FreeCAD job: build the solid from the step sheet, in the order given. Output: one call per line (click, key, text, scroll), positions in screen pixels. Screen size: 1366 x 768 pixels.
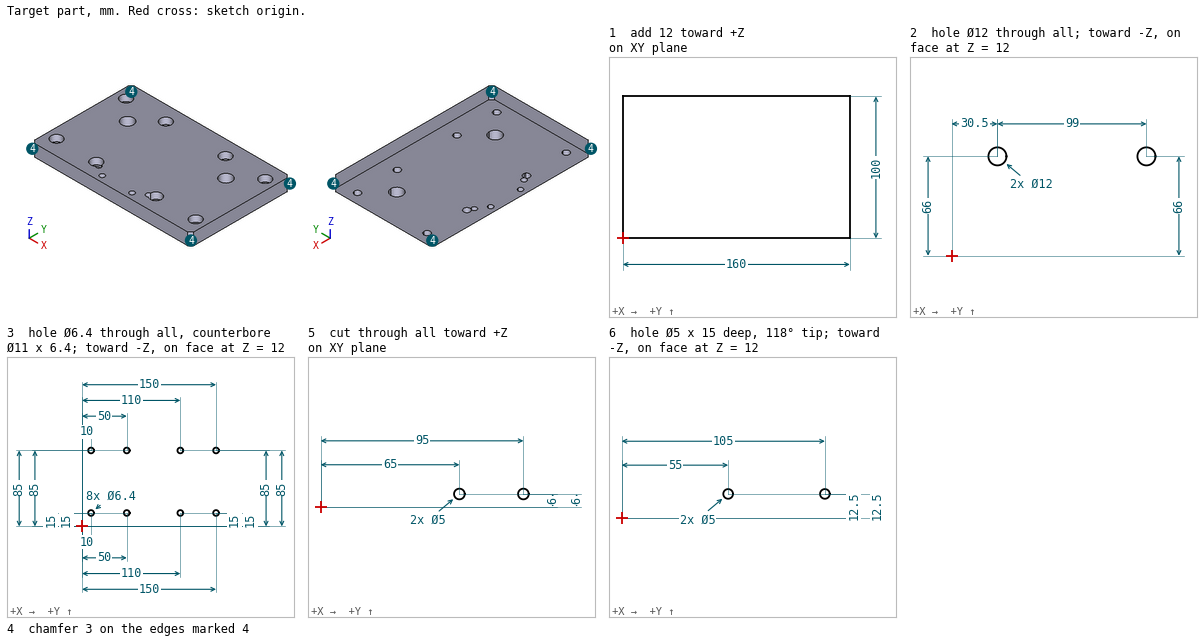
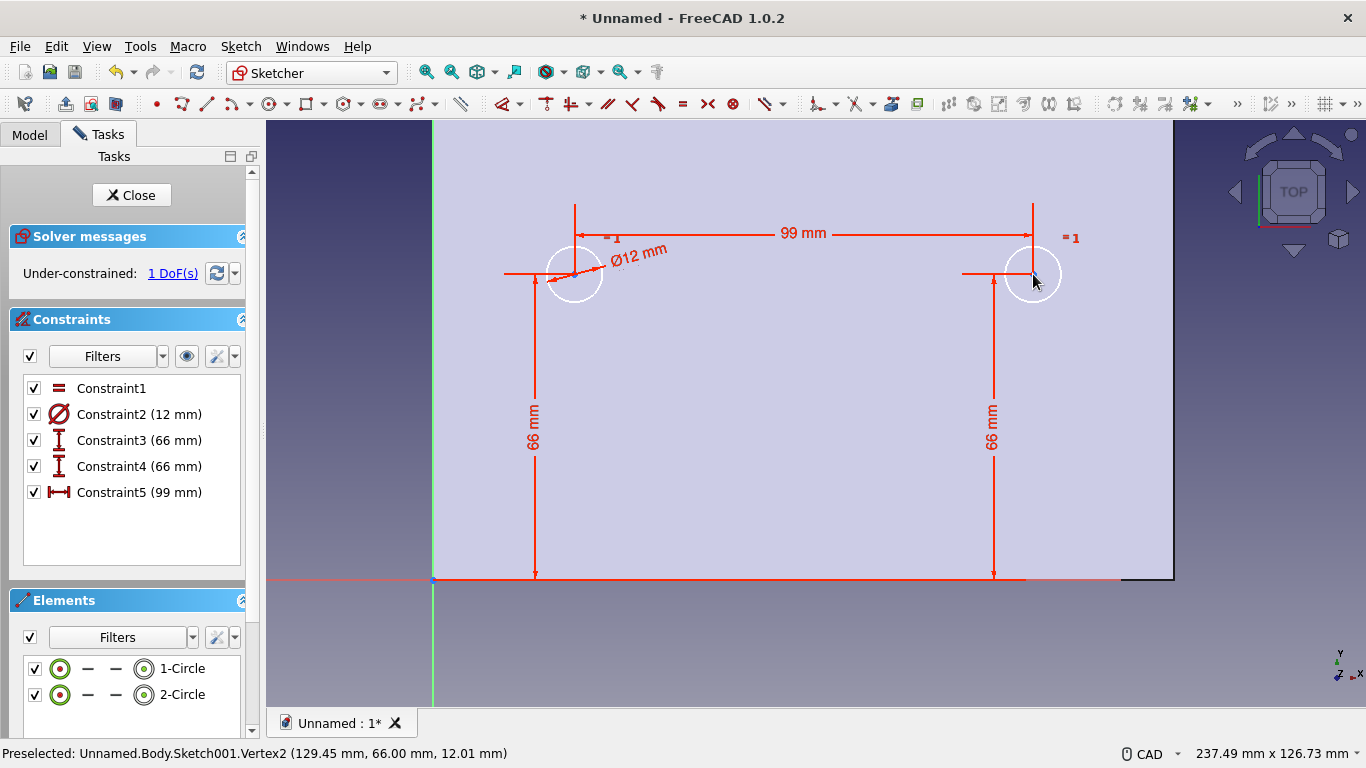
click(575, 274)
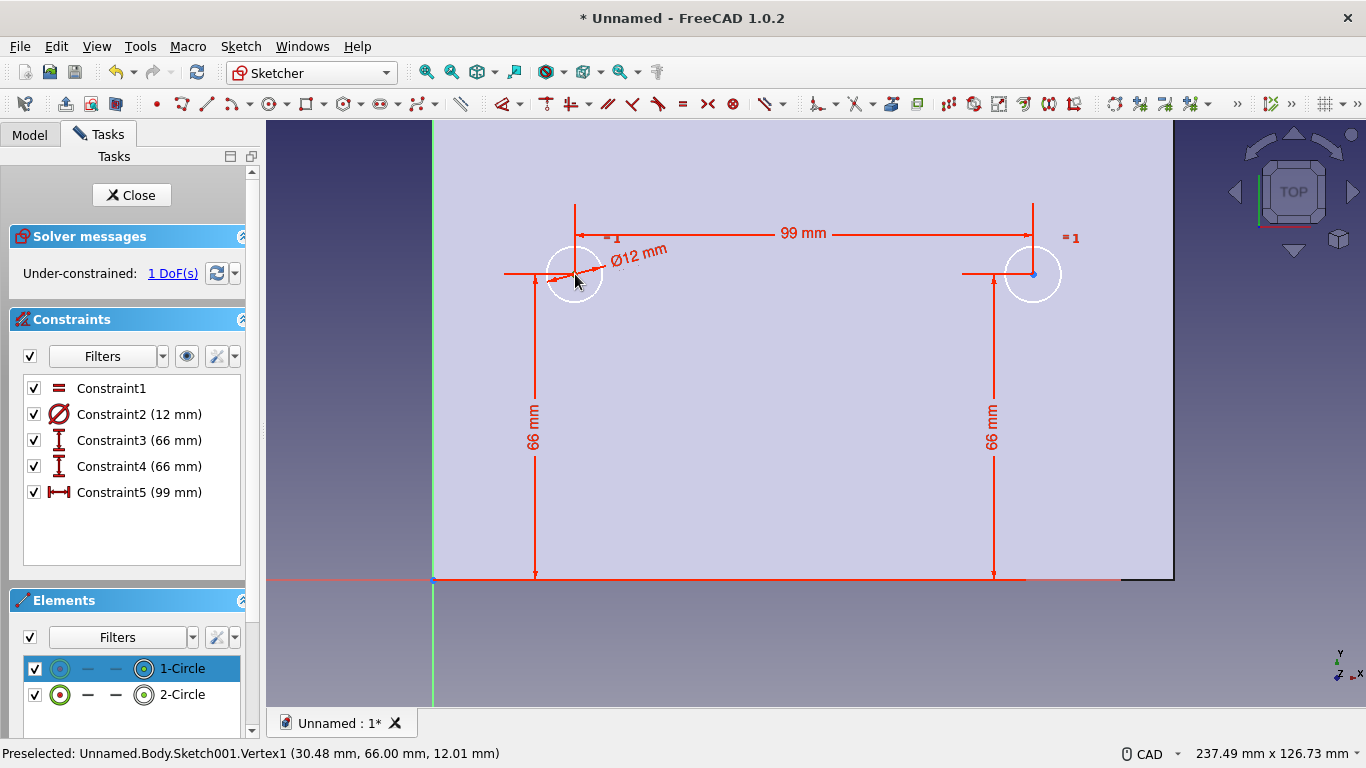
key(l)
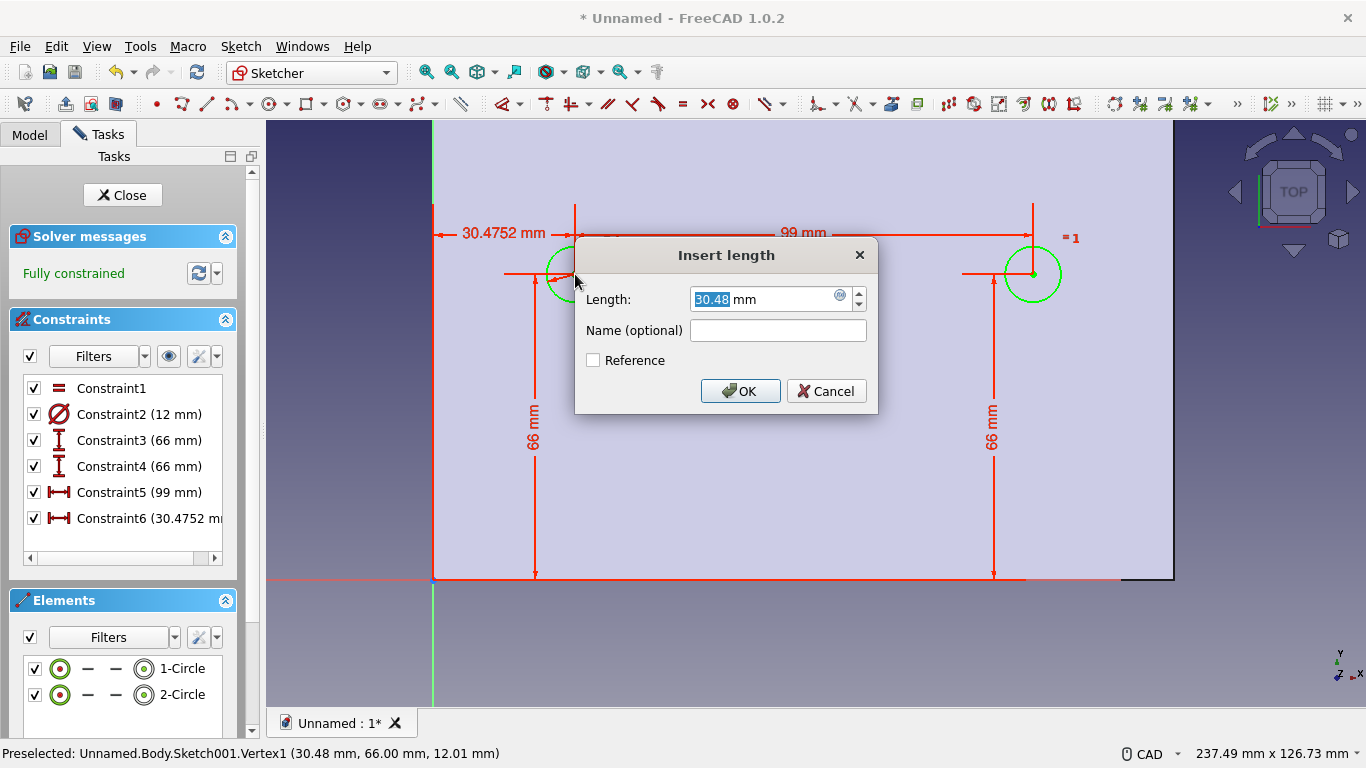
text(30.5)
key(Return)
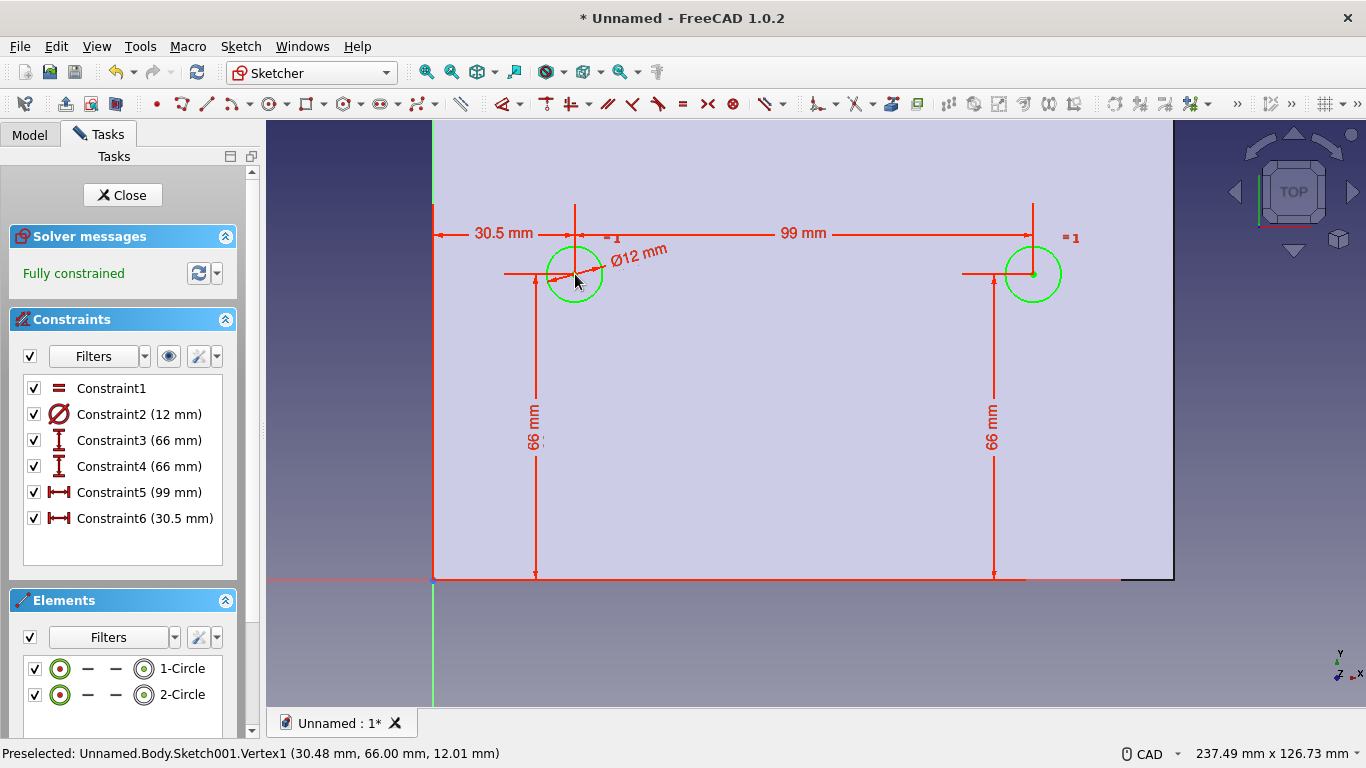
click(123, 195)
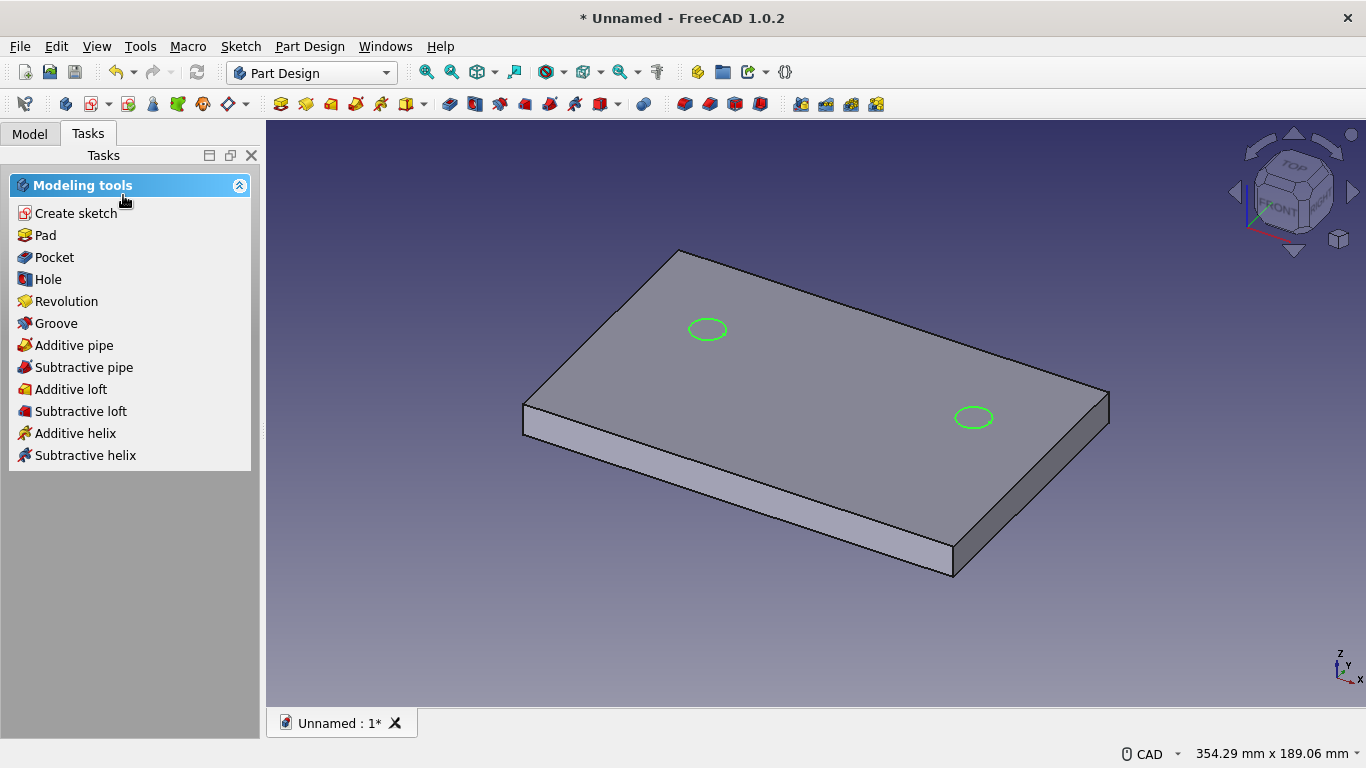
click(475, 104)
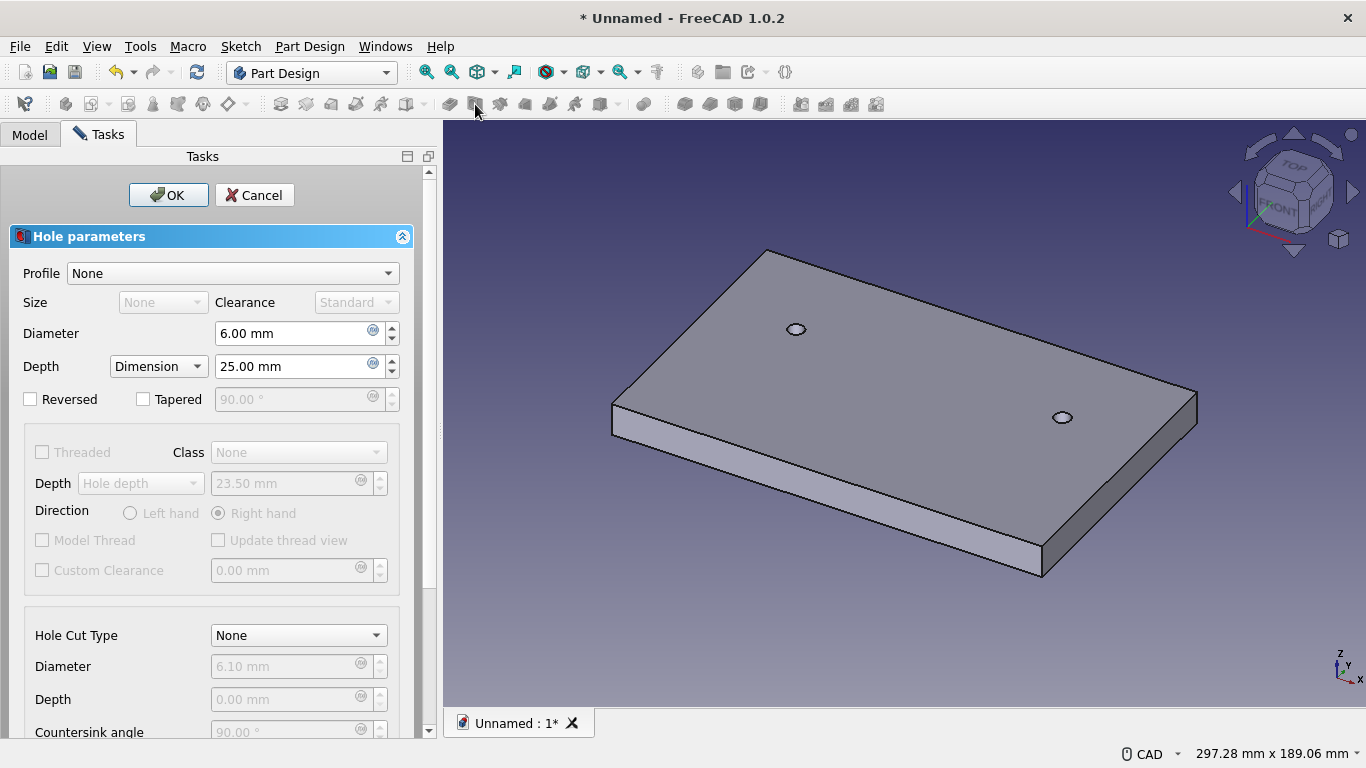
triple_click(300, 334)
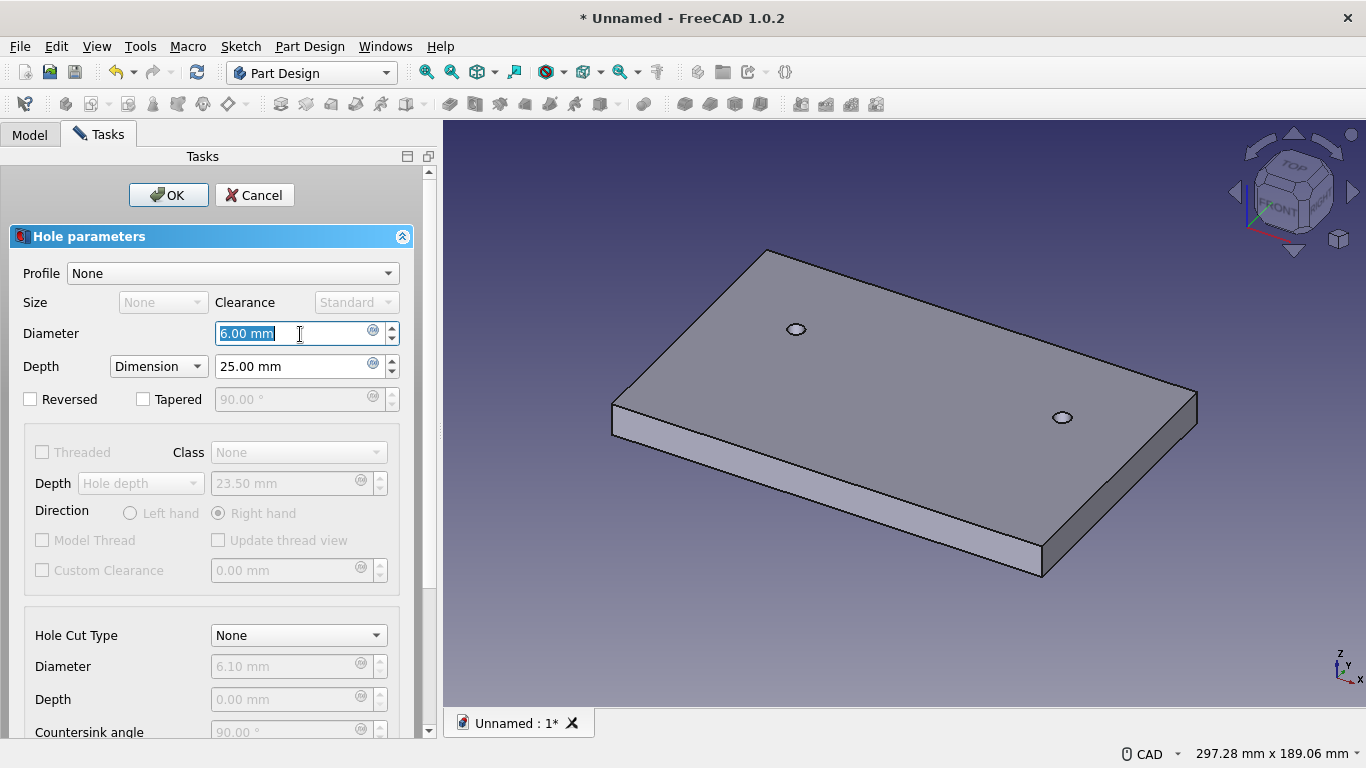
text(12)
key(Tab)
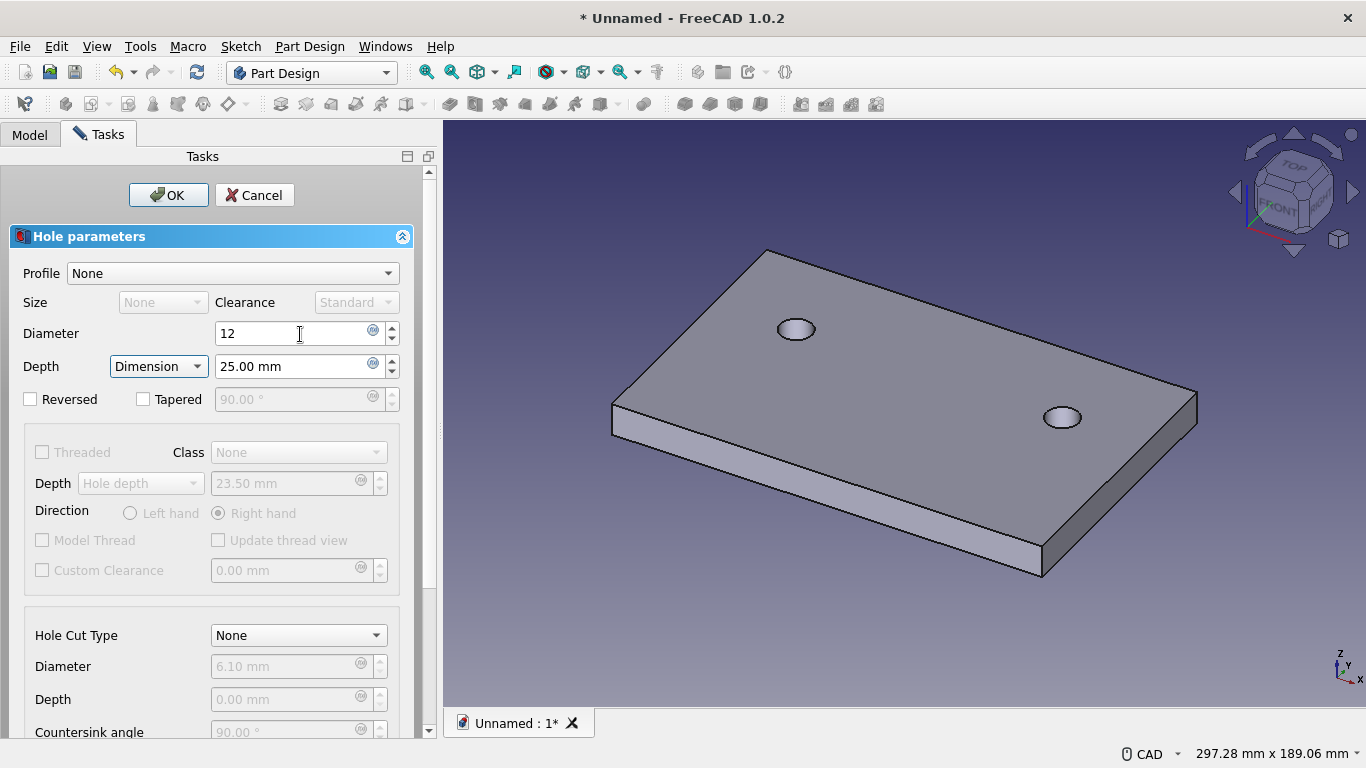
click(160, 366)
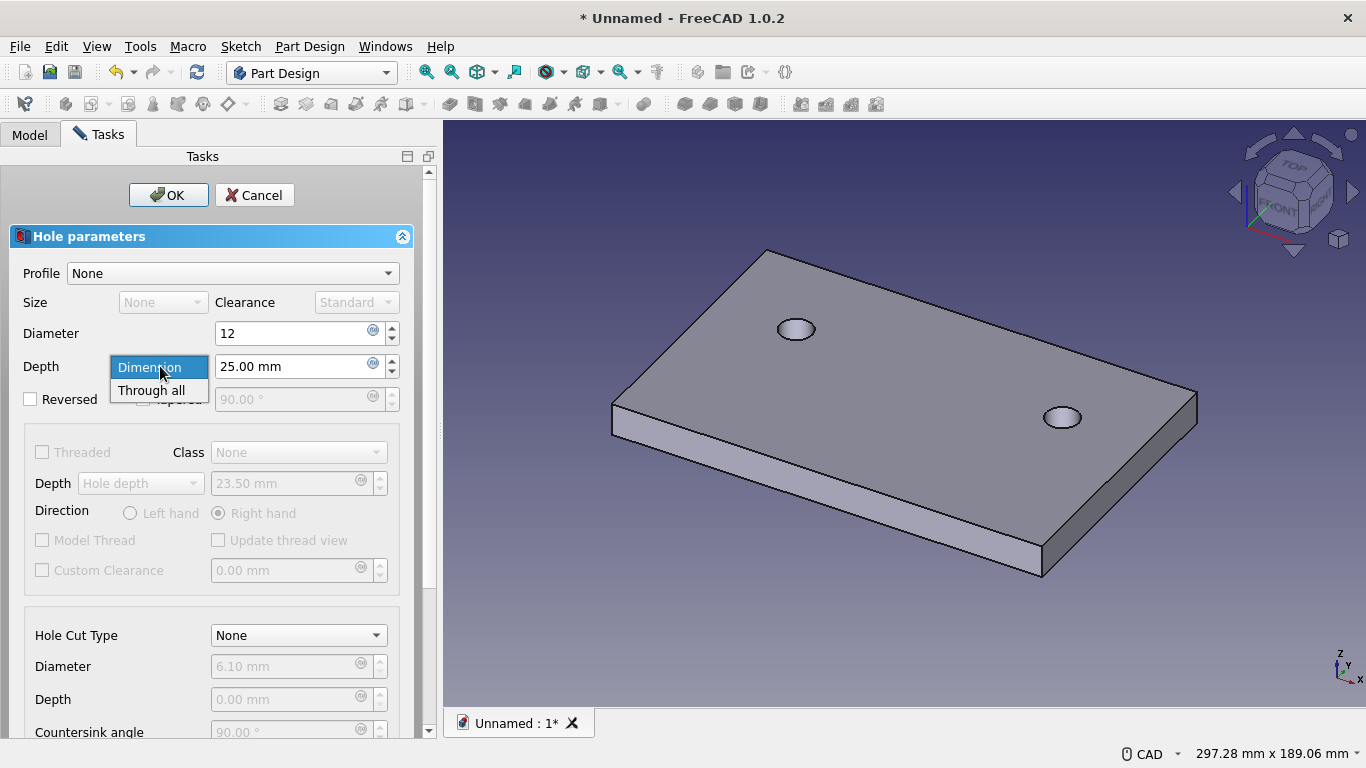
click(158, 390)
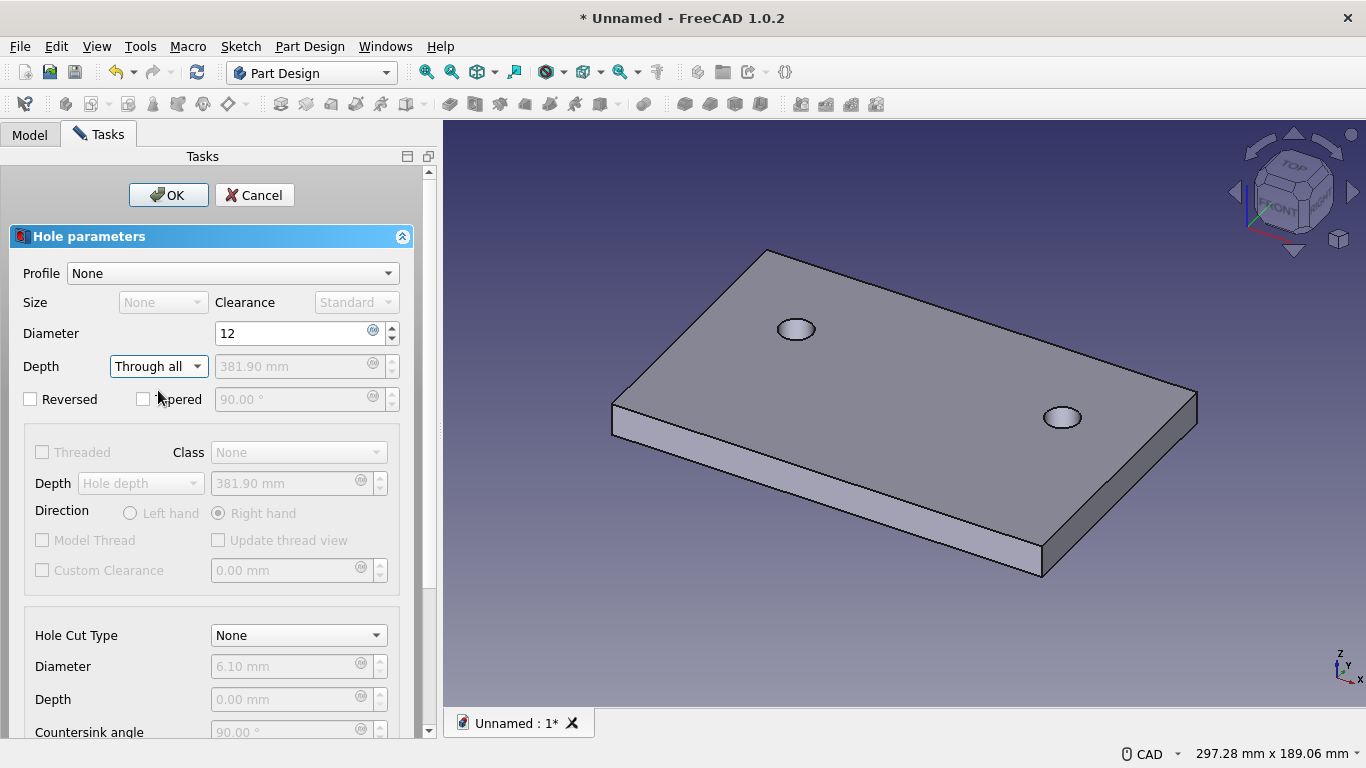
click(169, 195)